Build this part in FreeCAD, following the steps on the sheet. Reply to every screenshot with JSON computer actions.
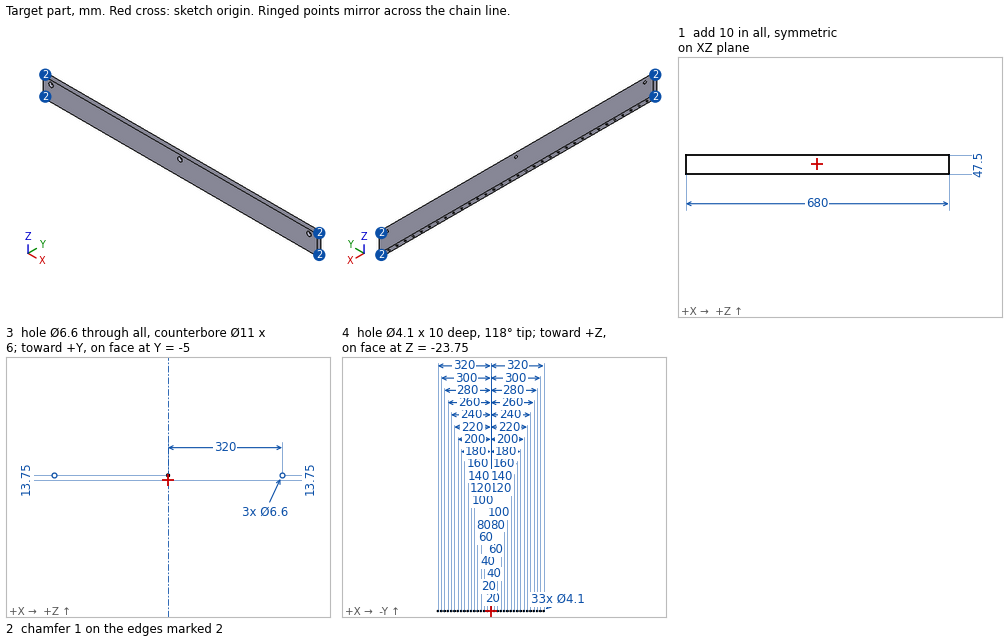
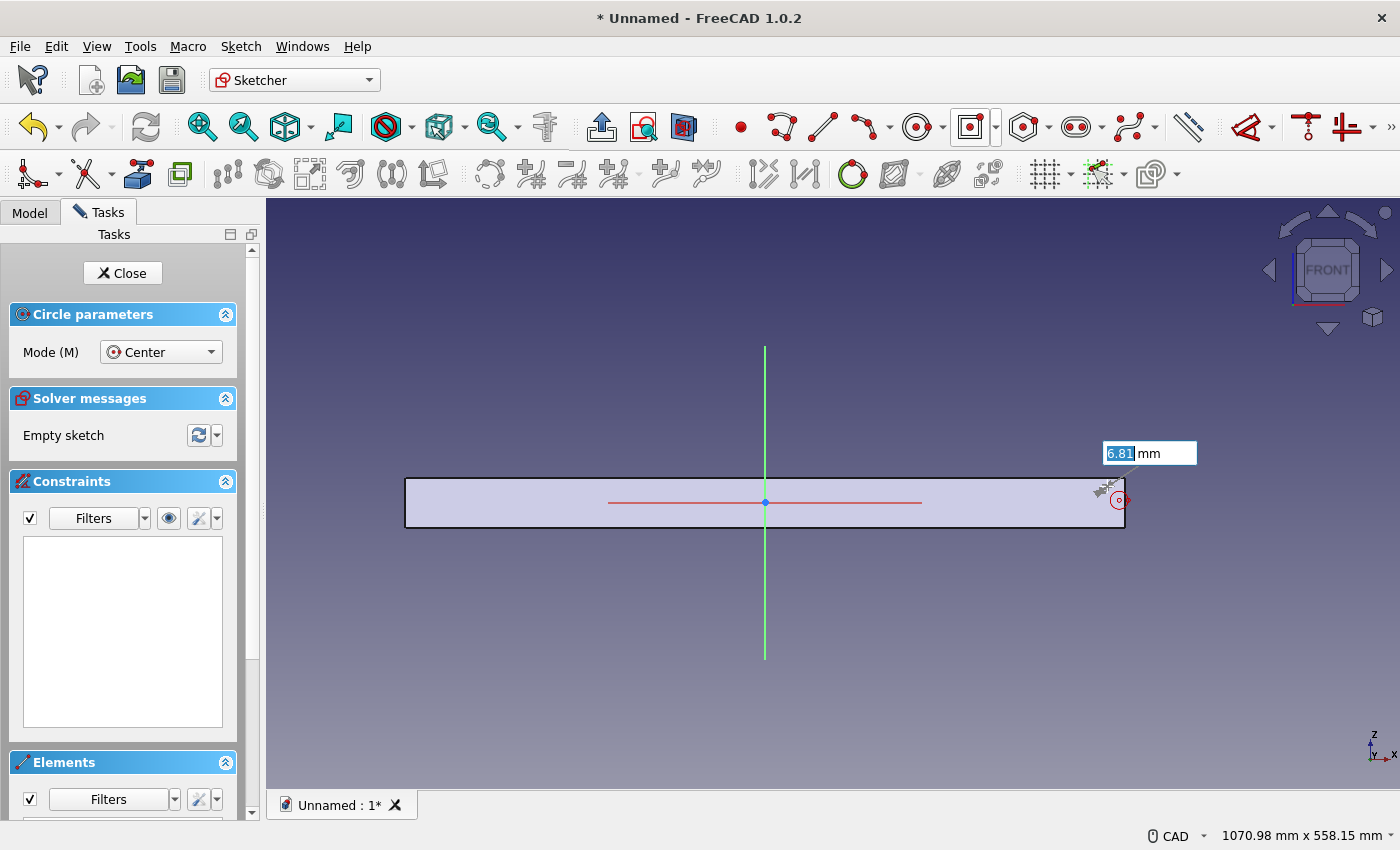
{"action": "type", "text": "6.6"}
{"action": "key", "text": "Return"}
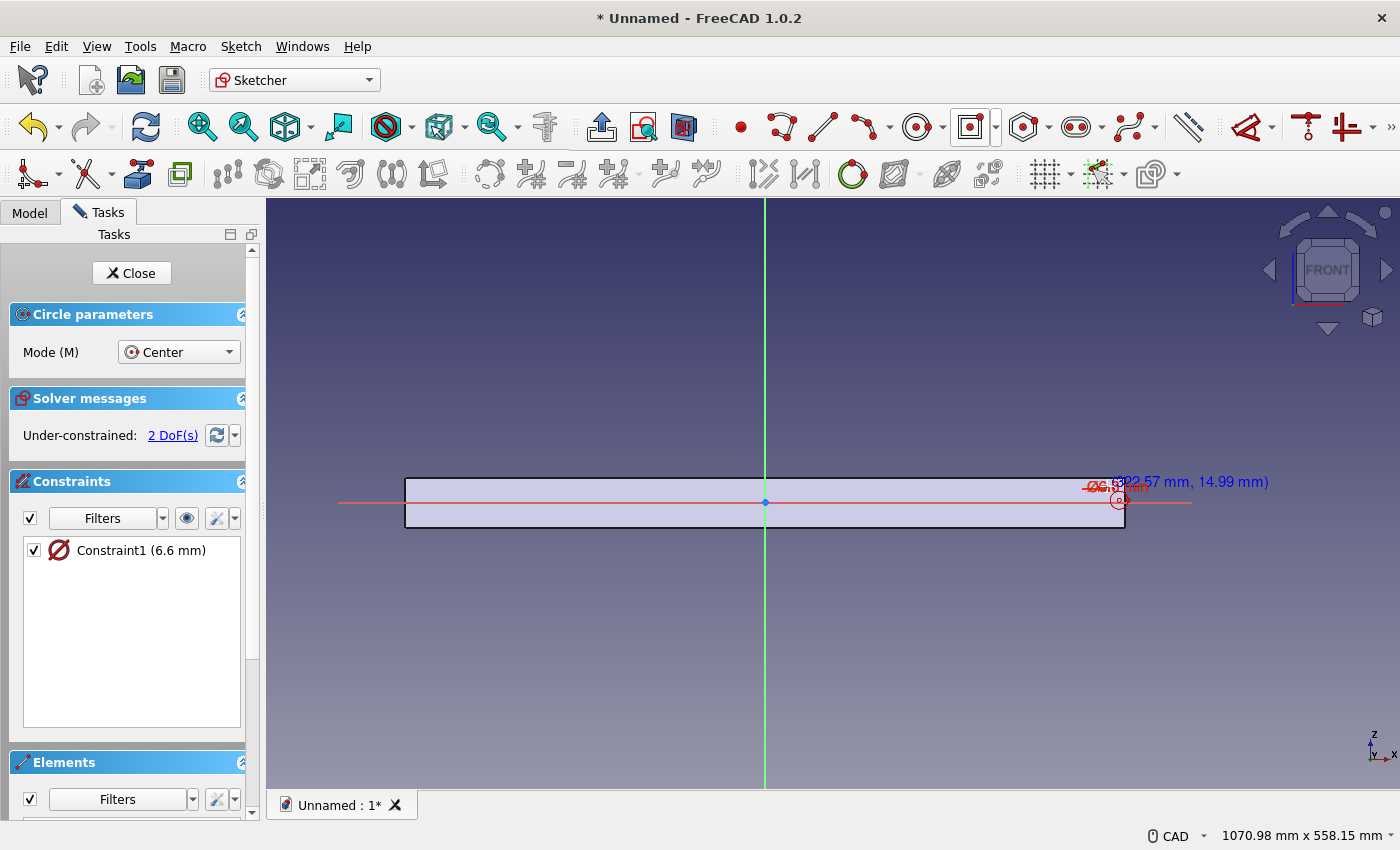
{"action": "scroll", "coordinate": [765, 488], "scroll_direction": "up", "scroll_amount": 10}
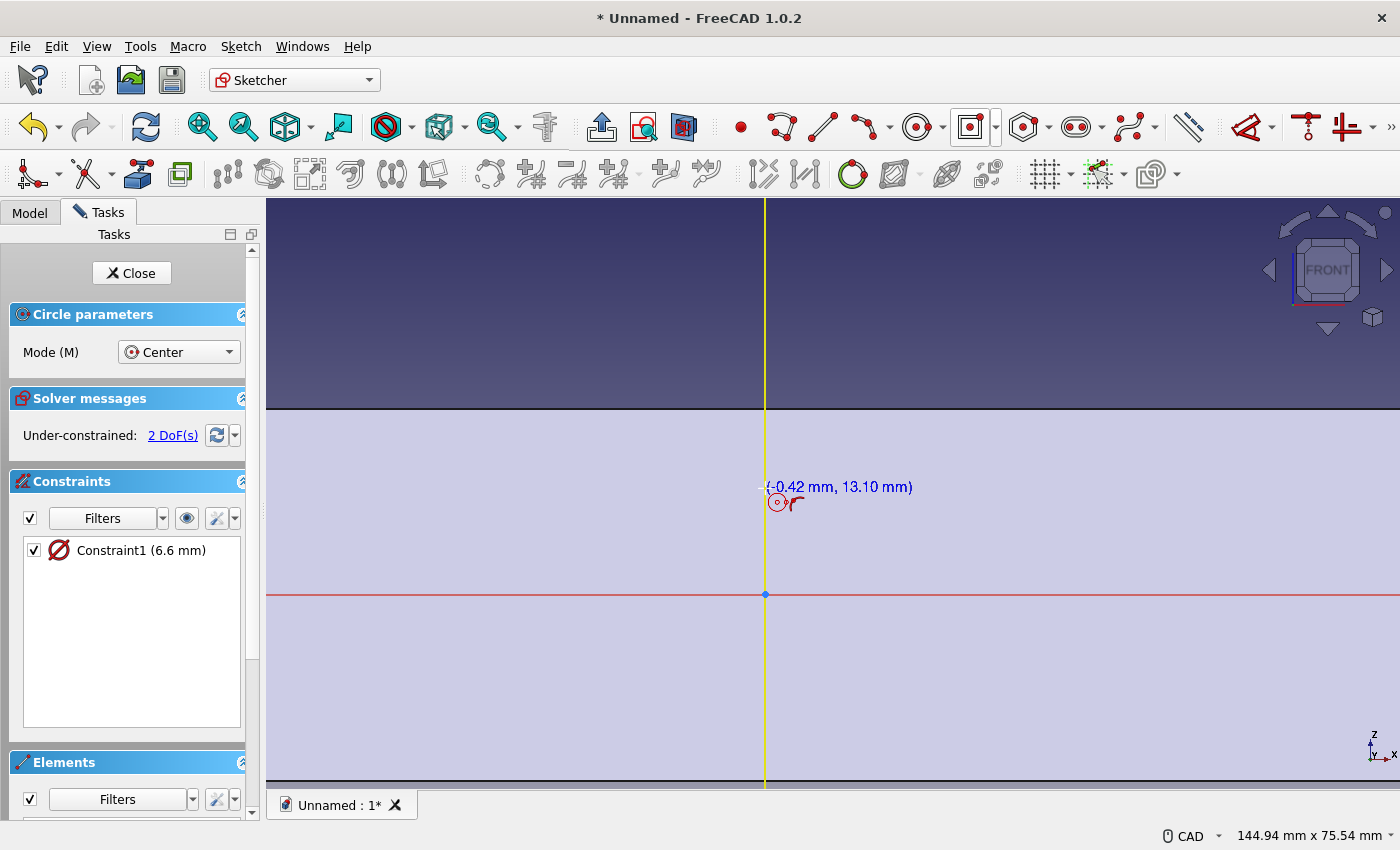
{"action": "scroll", "coordinate": [764, 488], "scroll_direction": "down", "scroll_amount": 10}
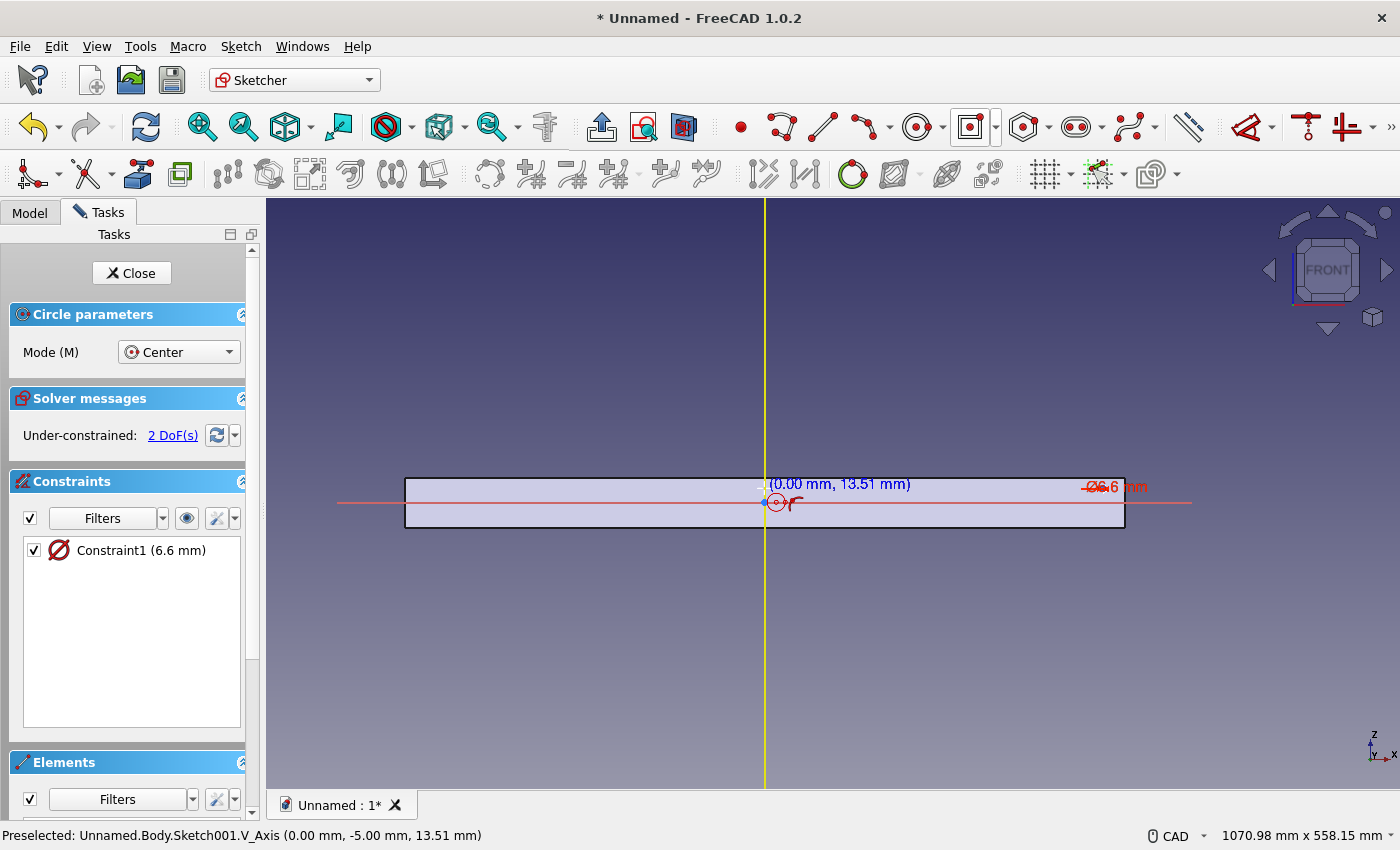
{"action": "left_click", "coordinate": [765, 488]}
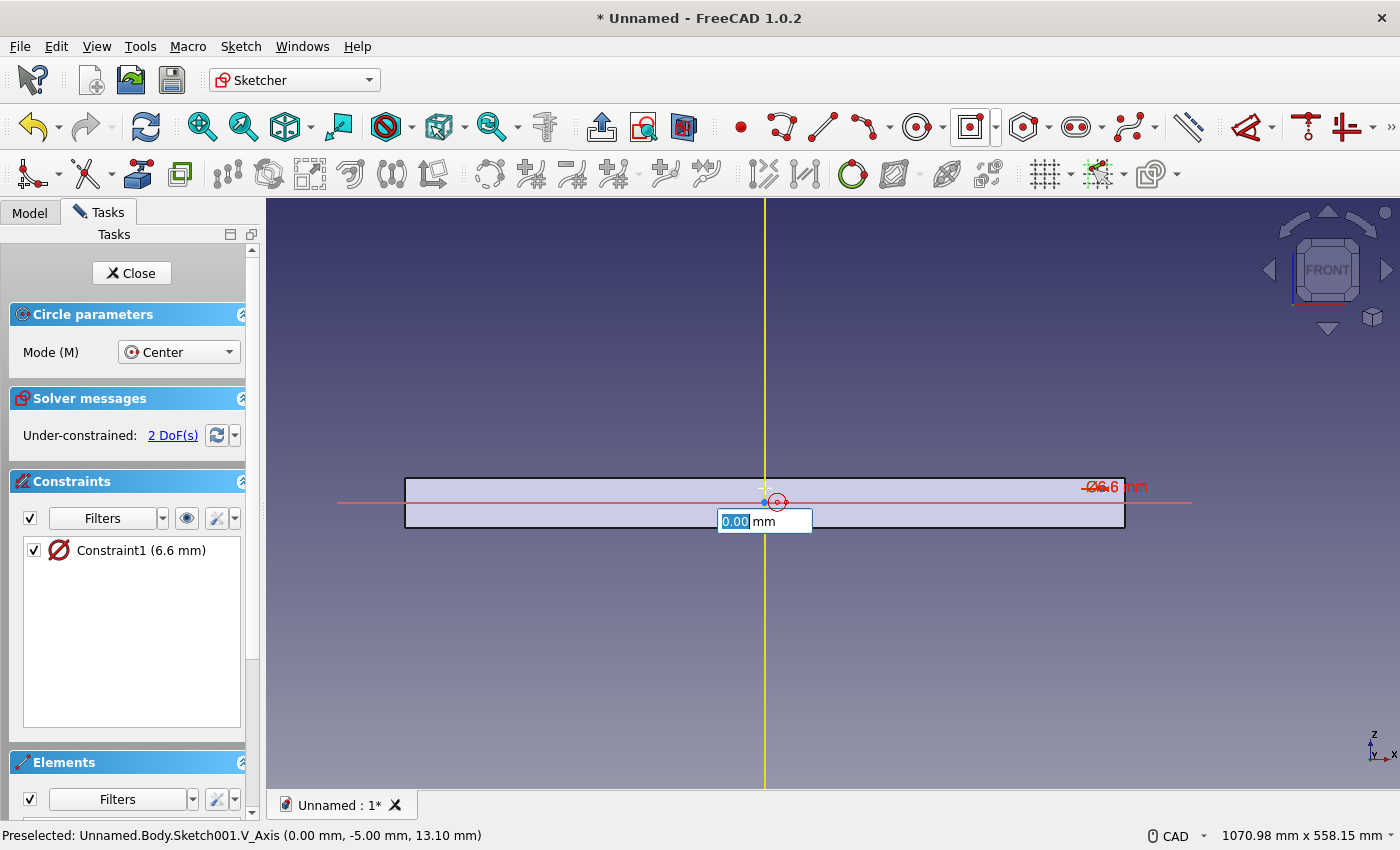
{"action": "scroll", "coordinate": [768, 487], "scroll_direction": "up", "scroll_amount": 8}
{"action": "mouse_move", "coordinate": [766, 486]}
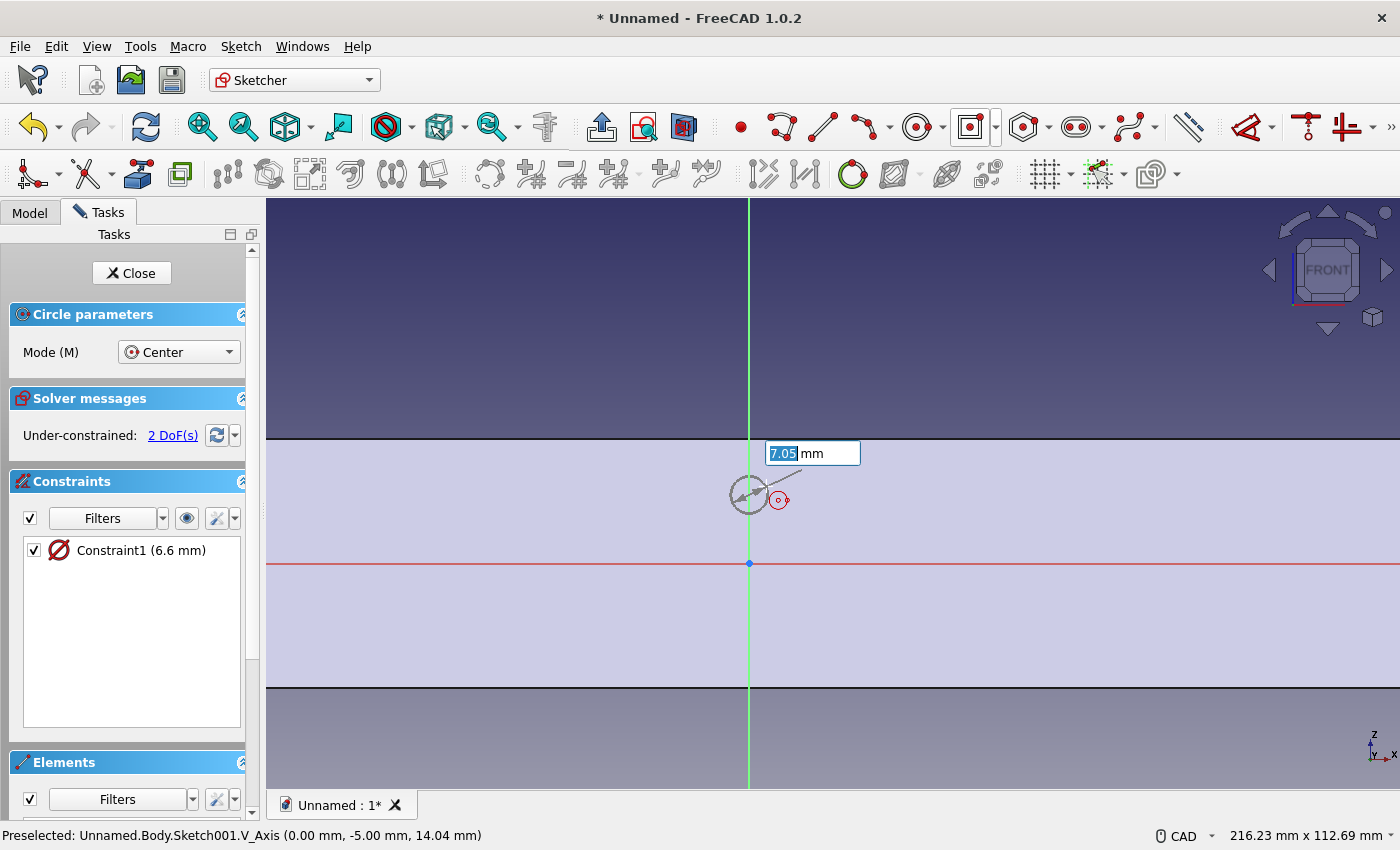
{"action": "type", "text": "6.6"}
{"action": "key", "text": "Return"}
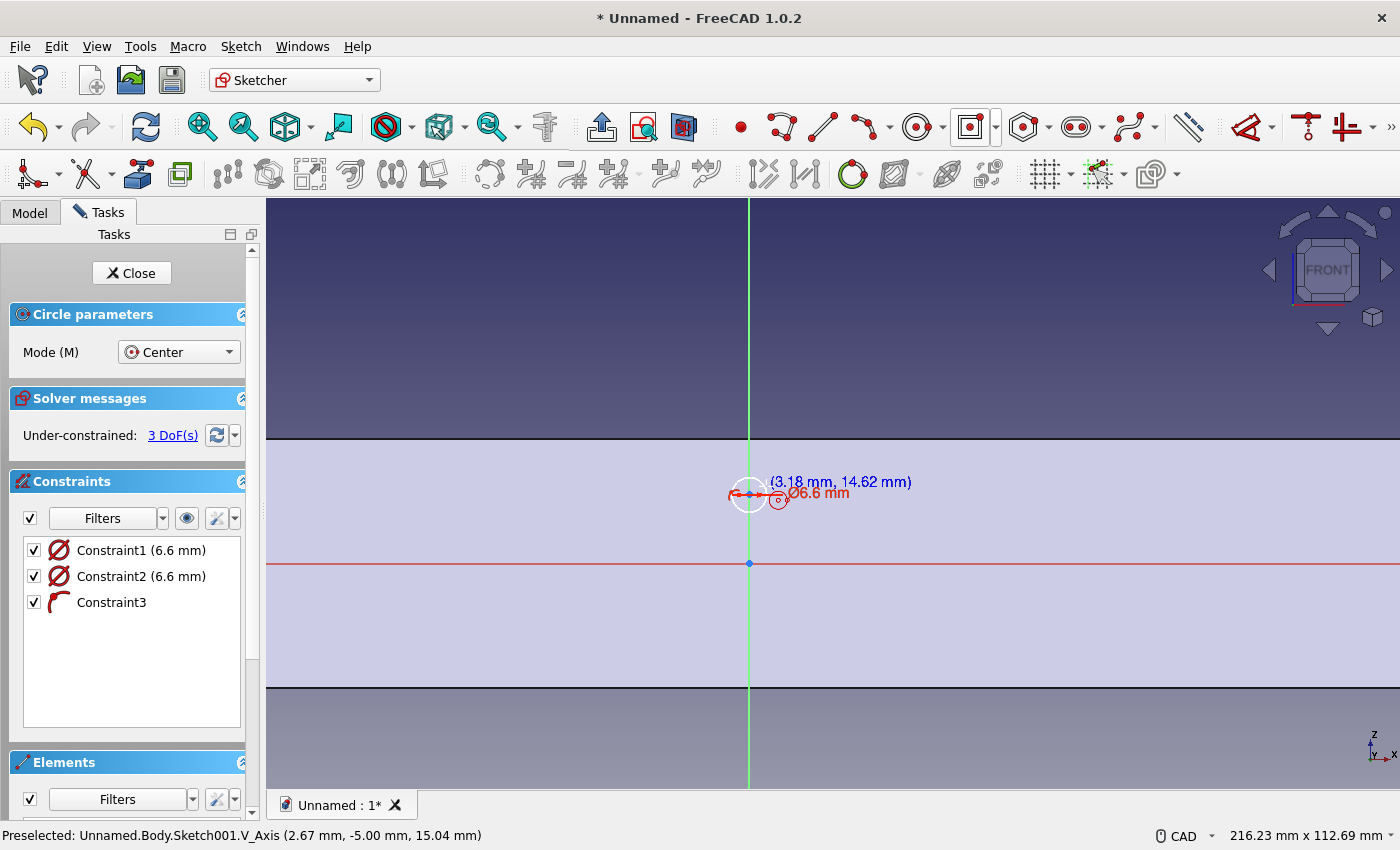
{"action": "scroll", "coordinate": [768, 487], "scroll_direction": "down", "scroll_amount": 8}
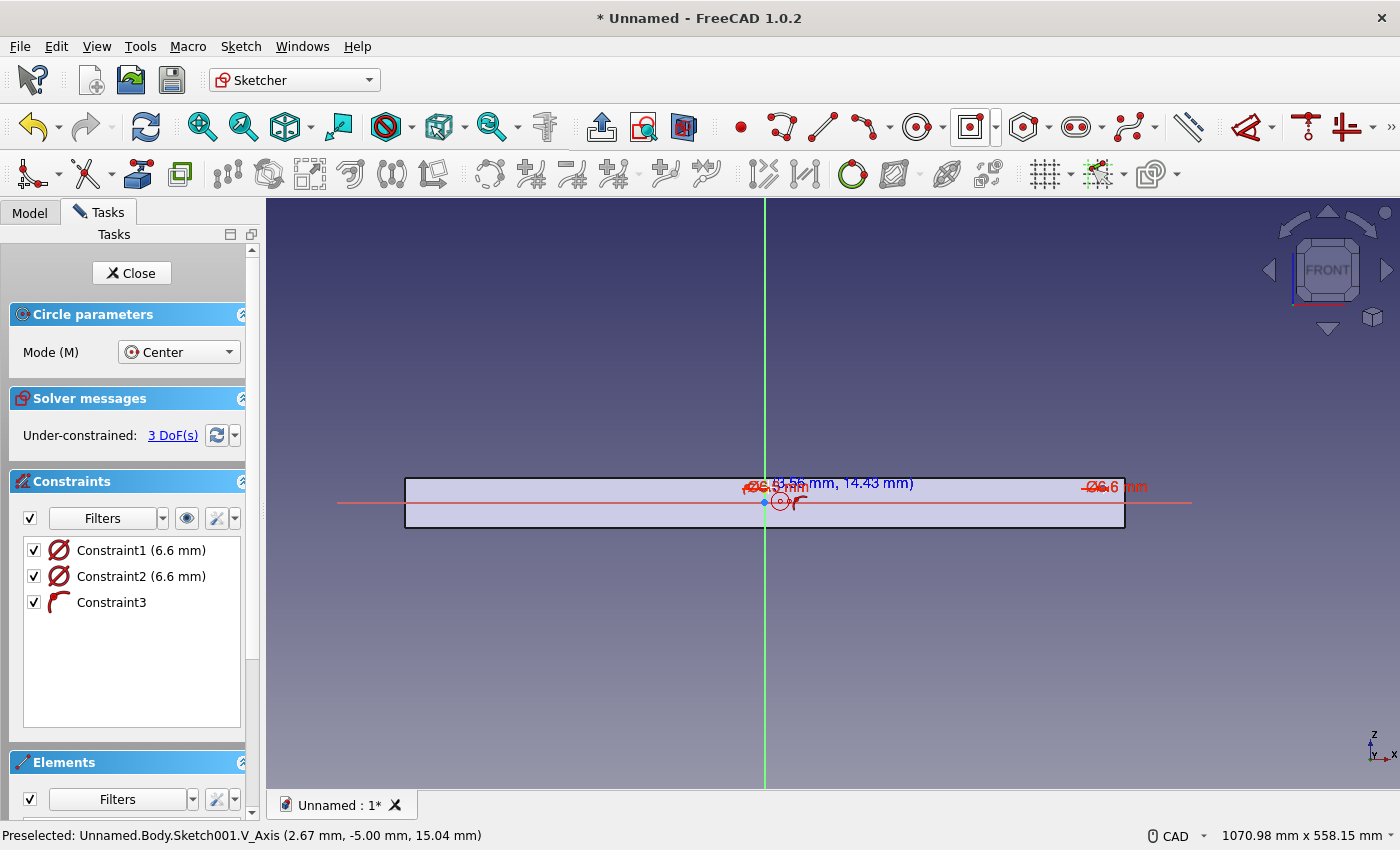
{"action": "scroll", "coordinate": [426, 488], "scroll_direction": "up", "scroll_amount": 10}